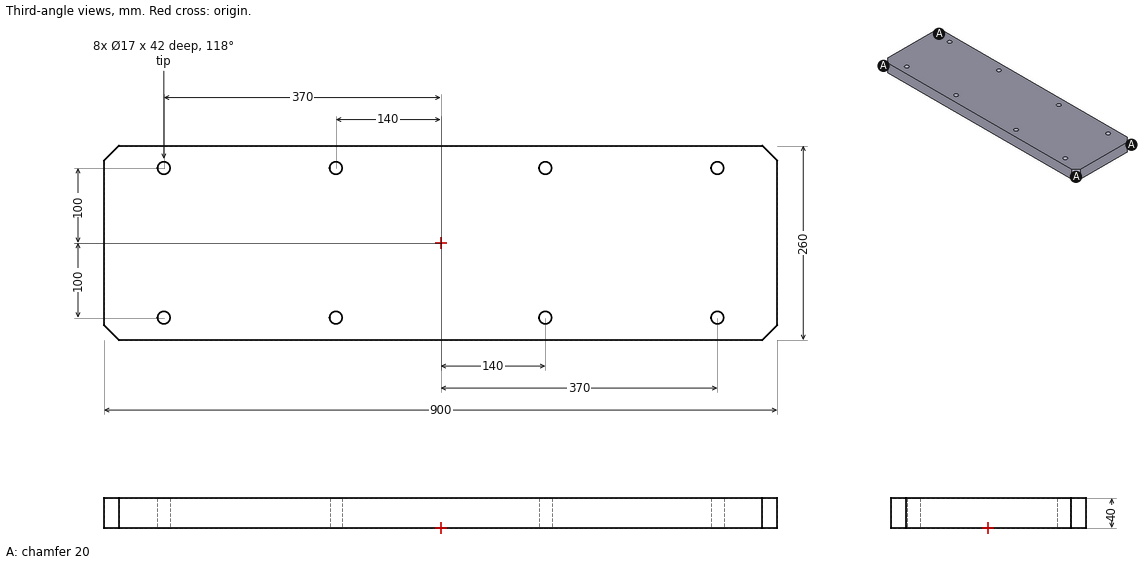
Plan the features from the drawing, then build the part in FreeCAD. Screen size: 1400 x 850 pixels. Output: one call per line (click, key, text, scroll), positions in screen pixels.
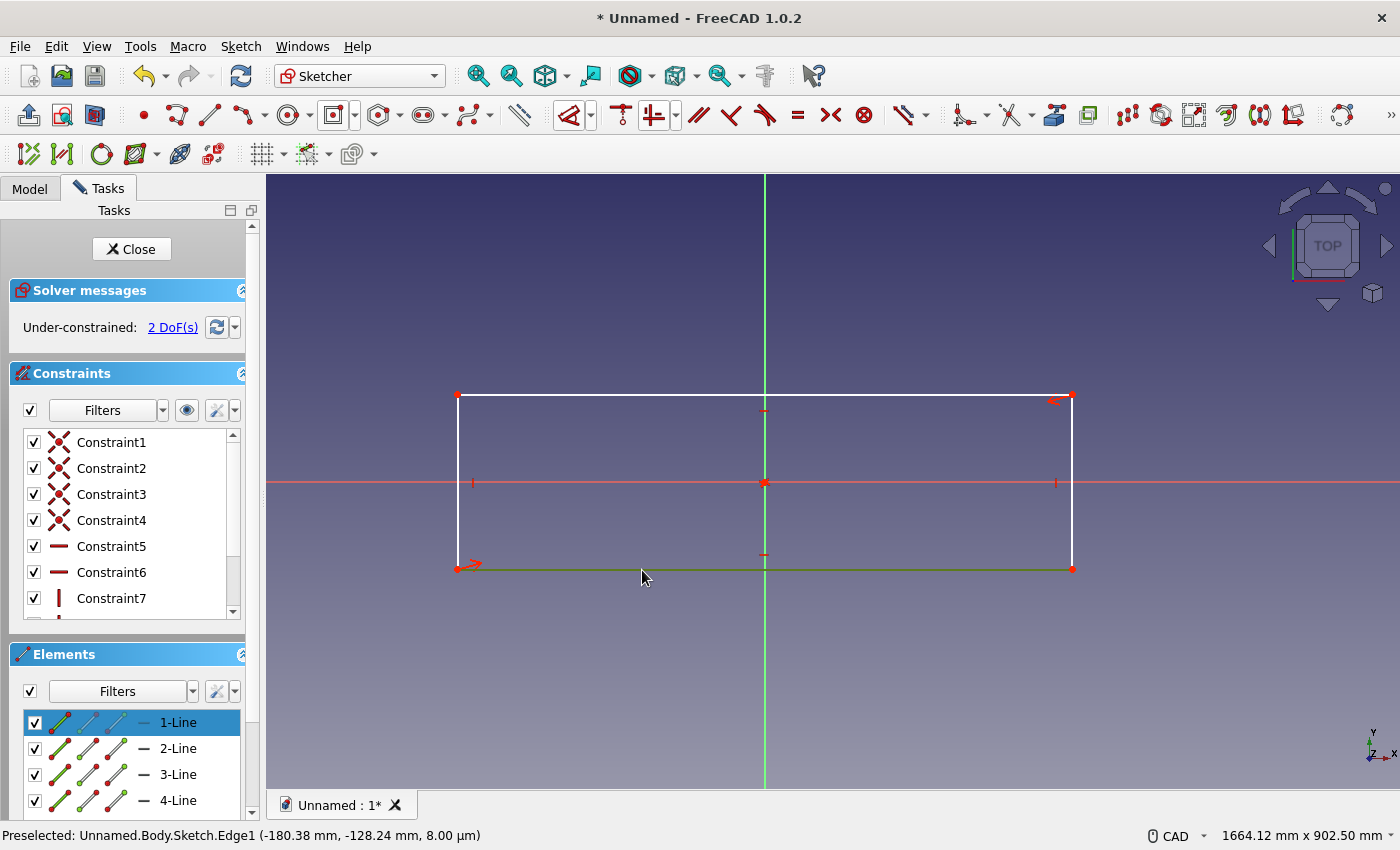
click(590, 116)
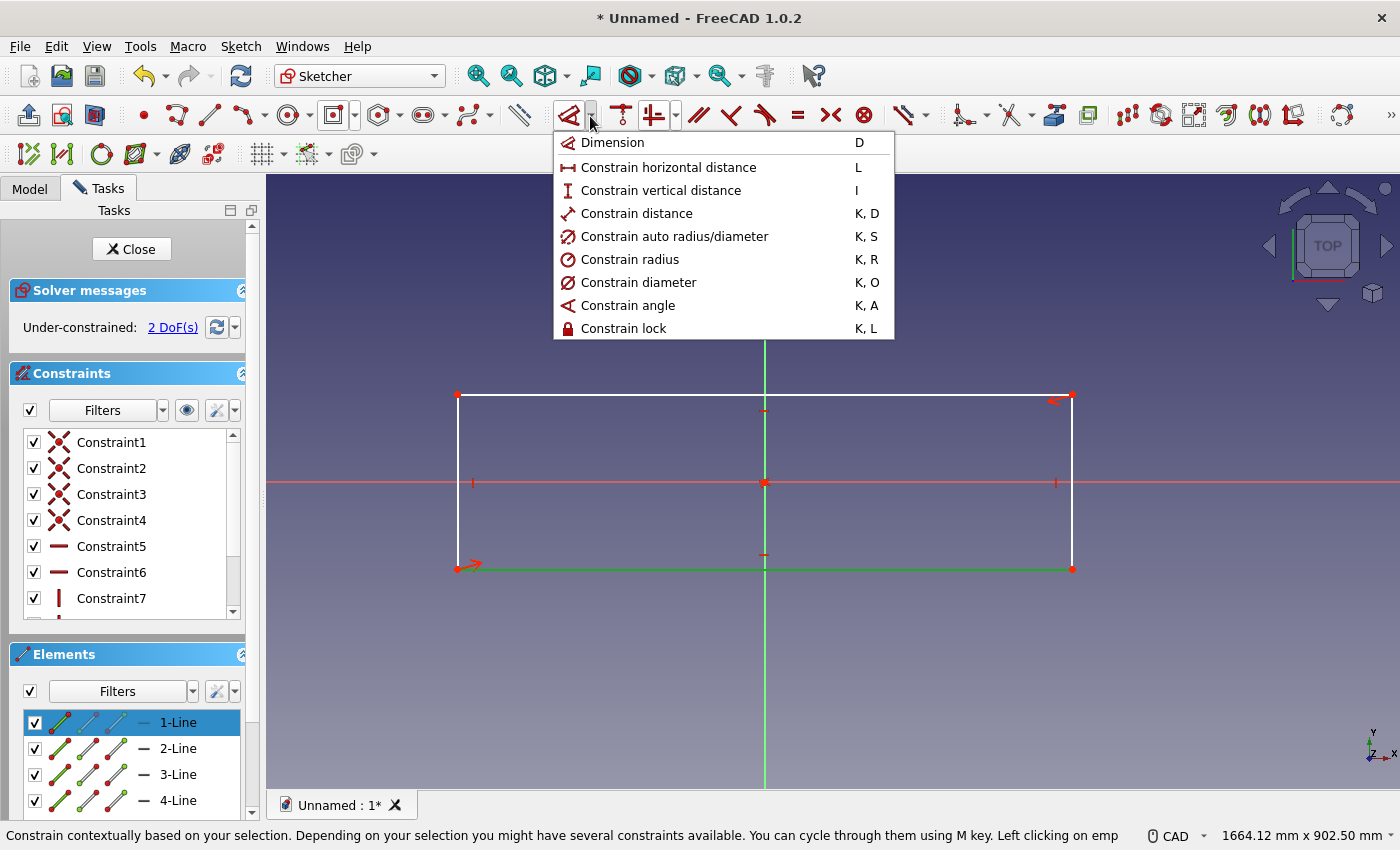
click(724, 168)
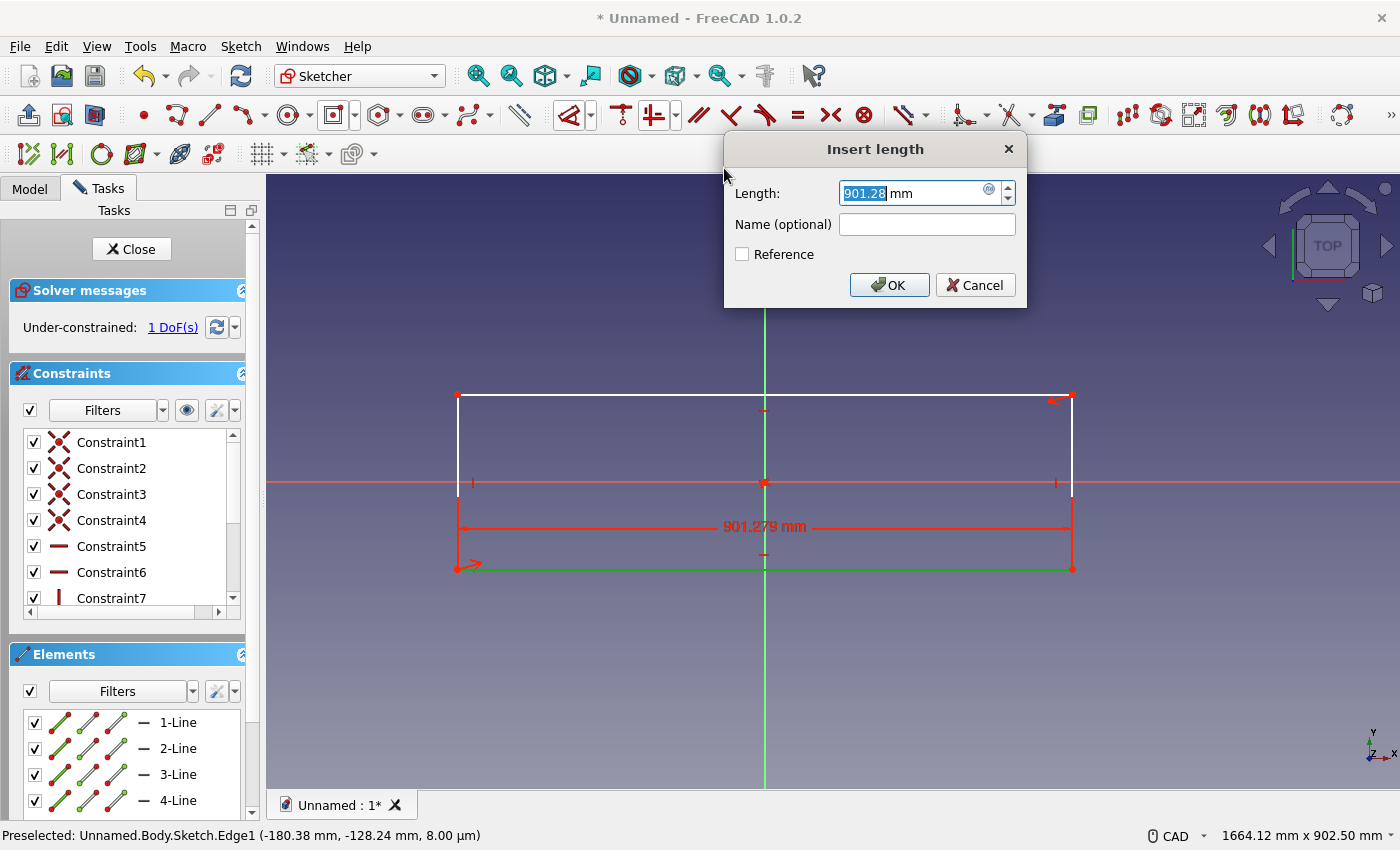
text(900)
key(Return)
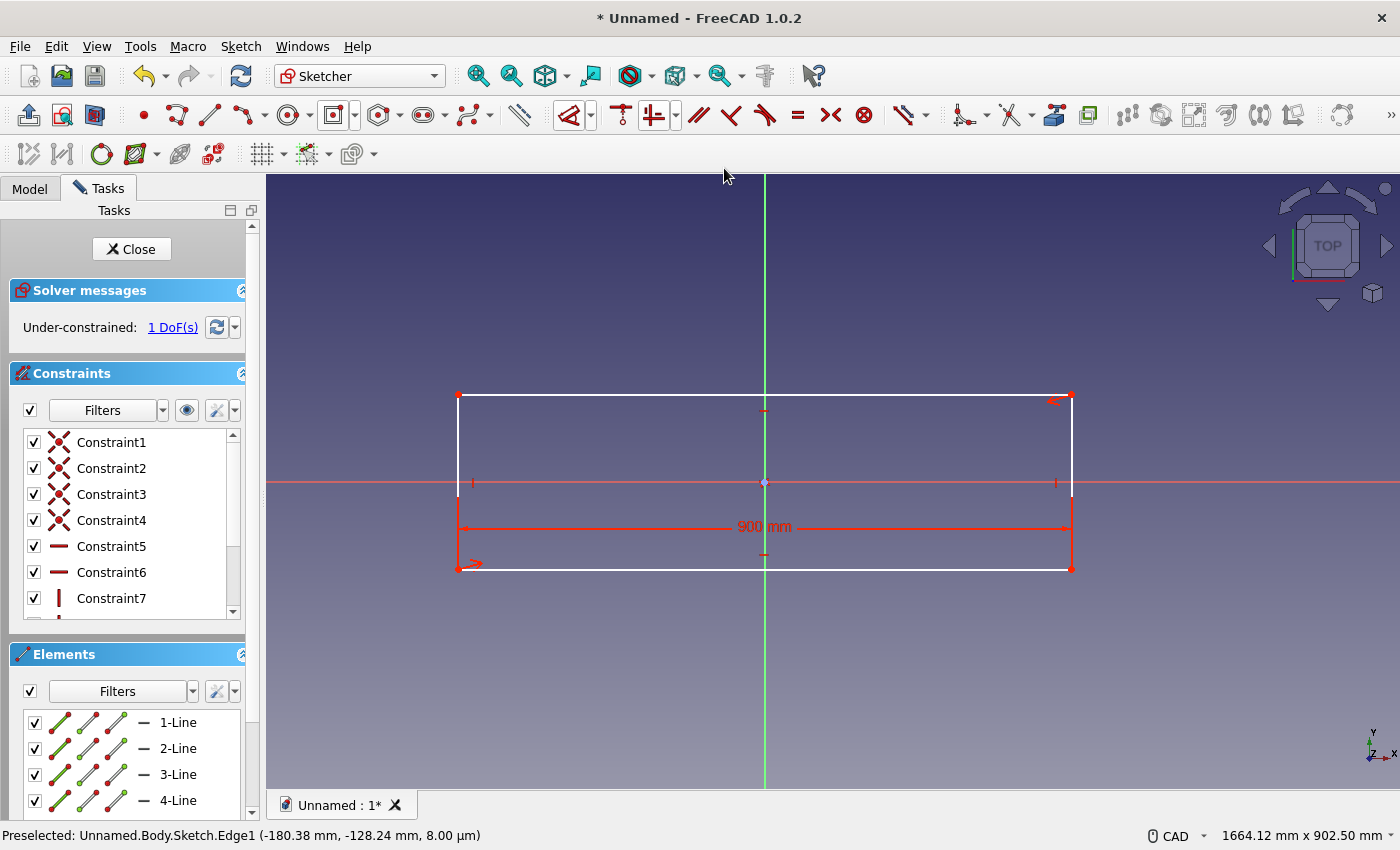
click(1072, 517)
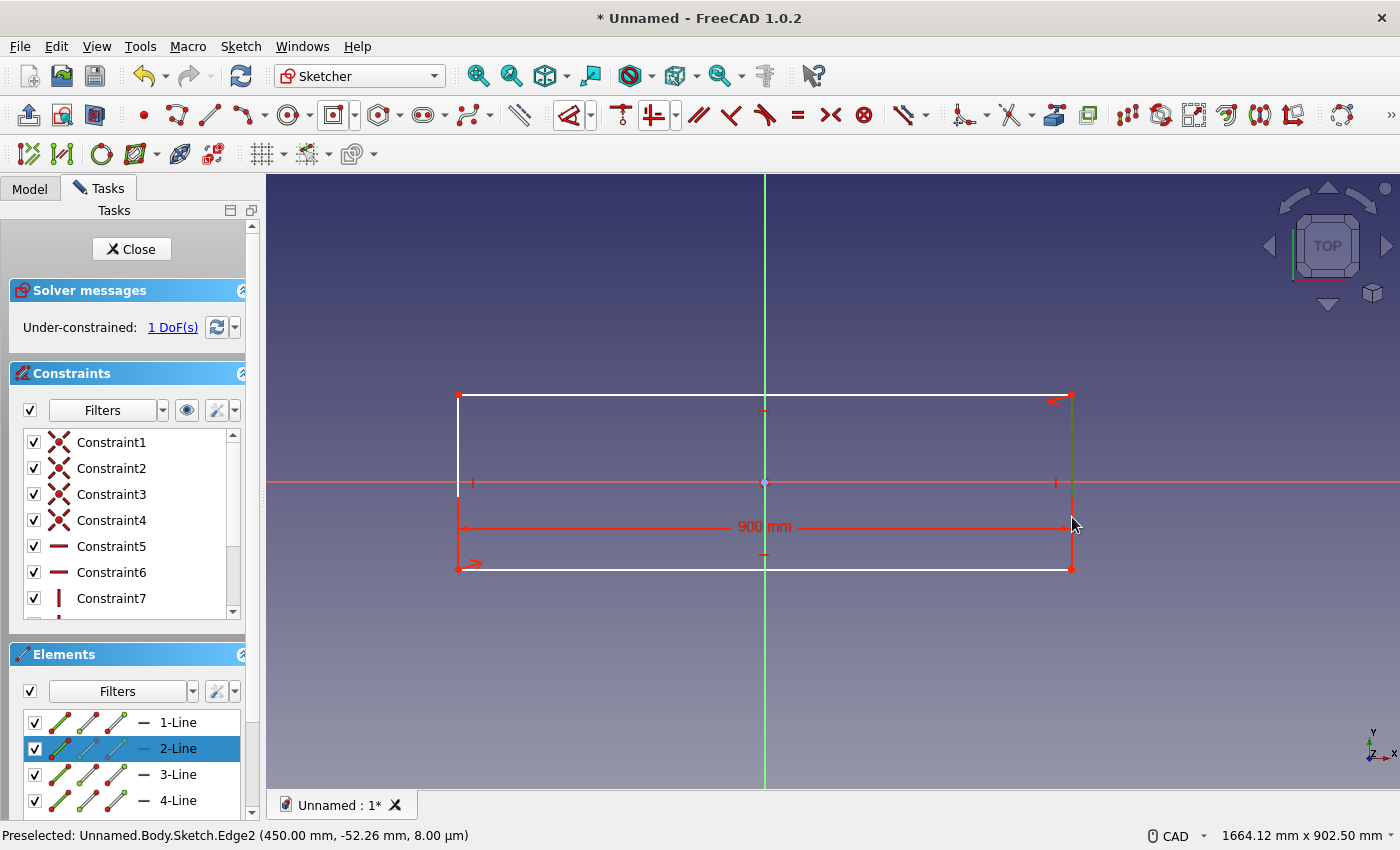
key(i)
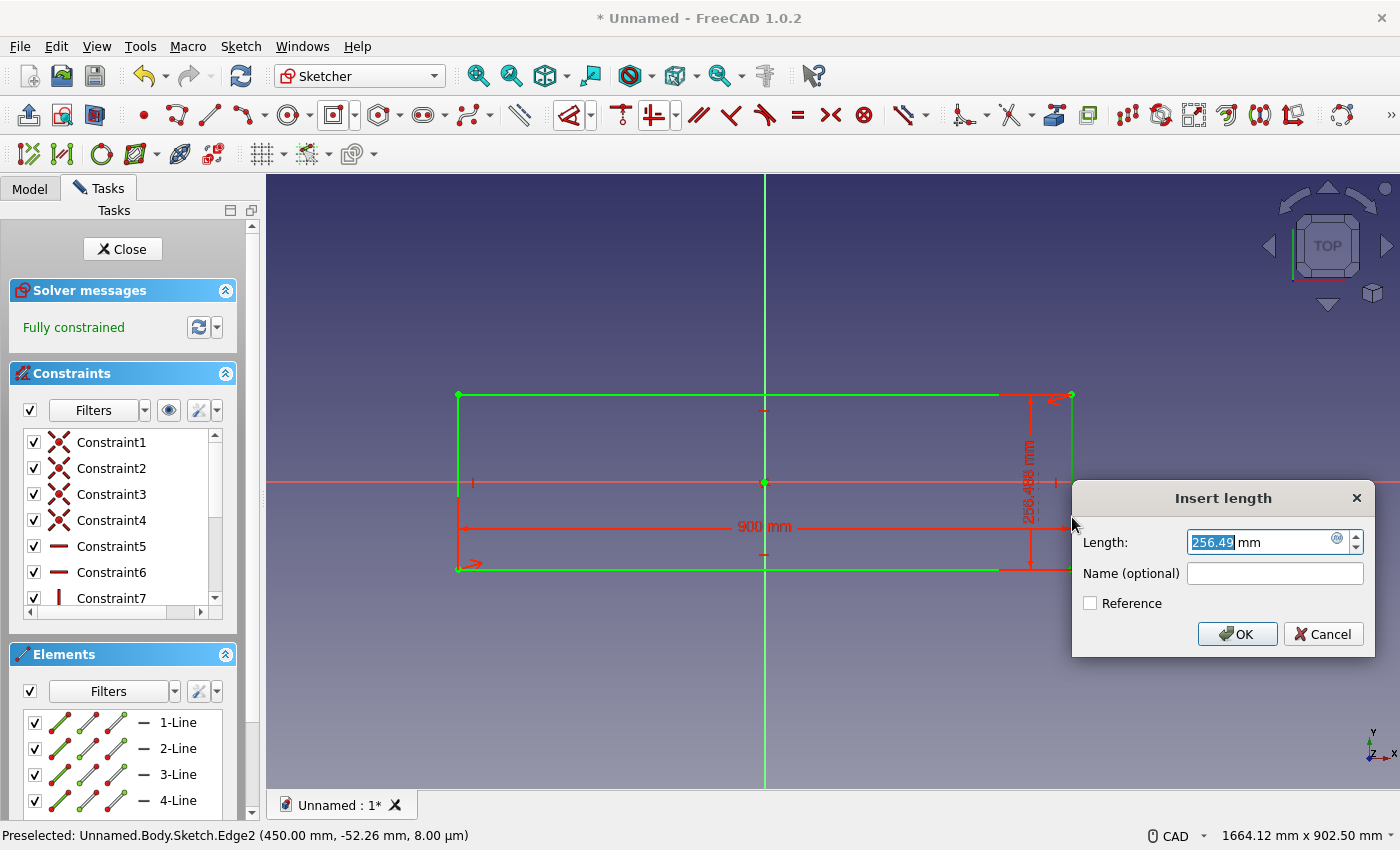
text(260)
key(Return)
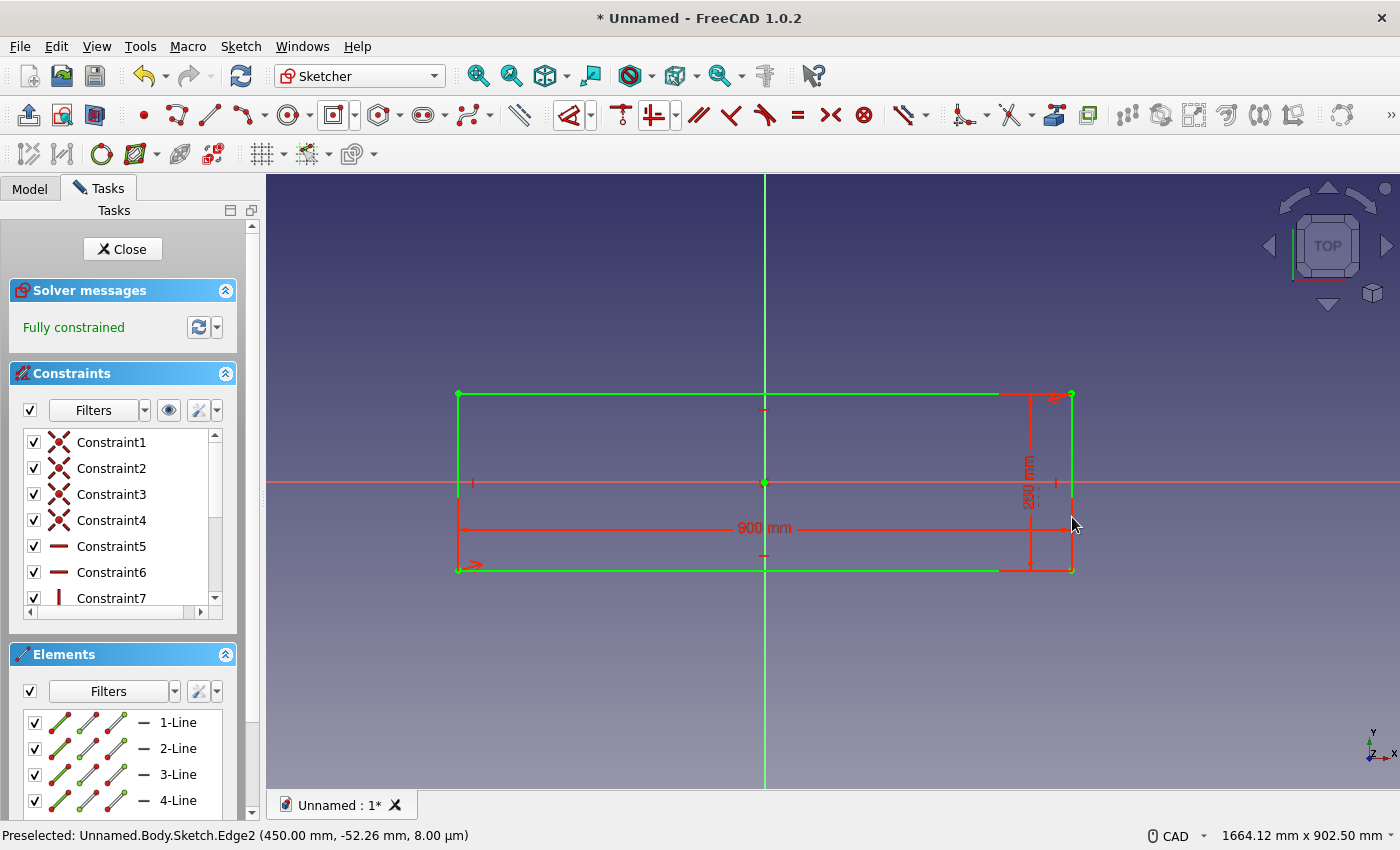
click(123, 249)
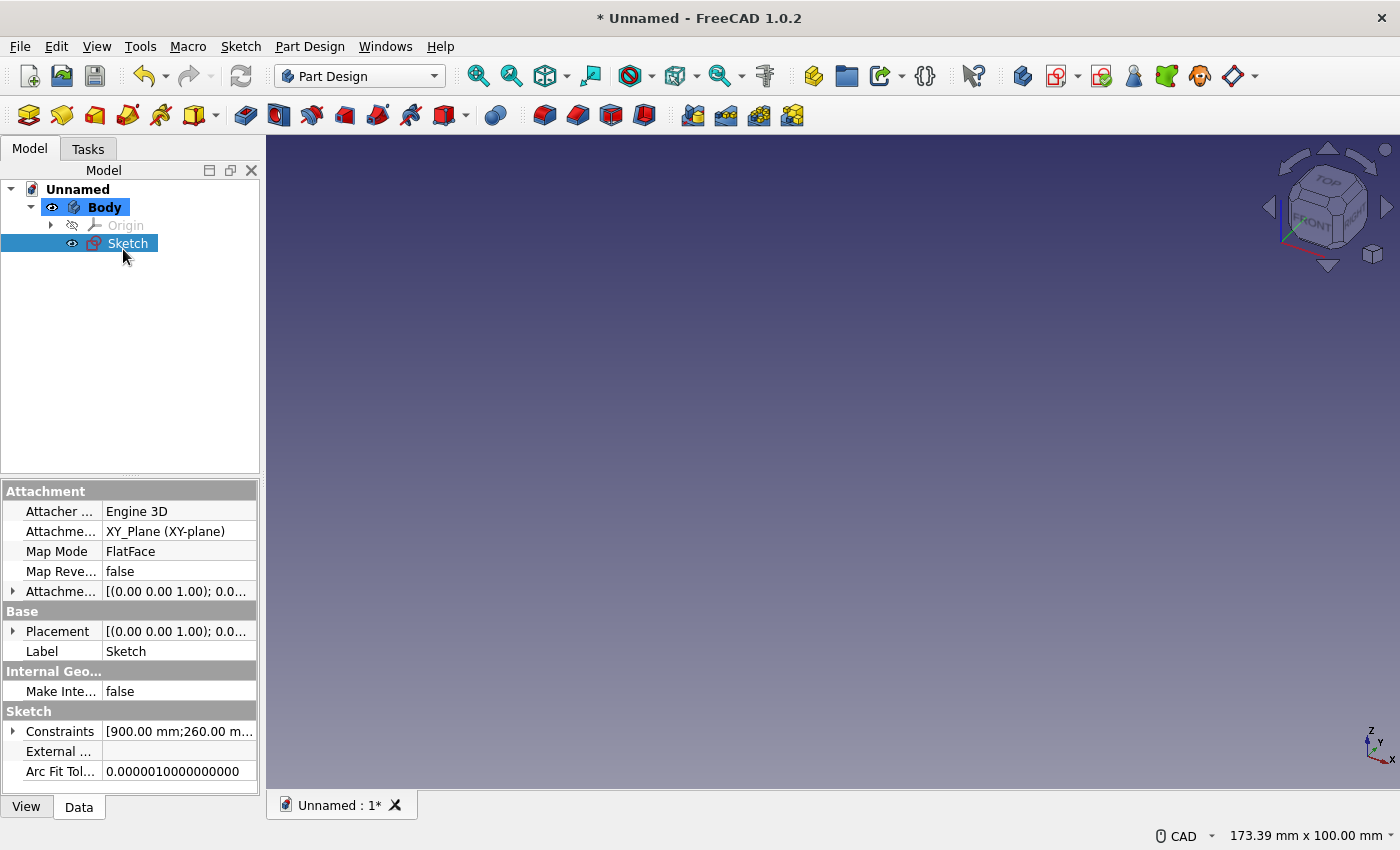
click(29, 116)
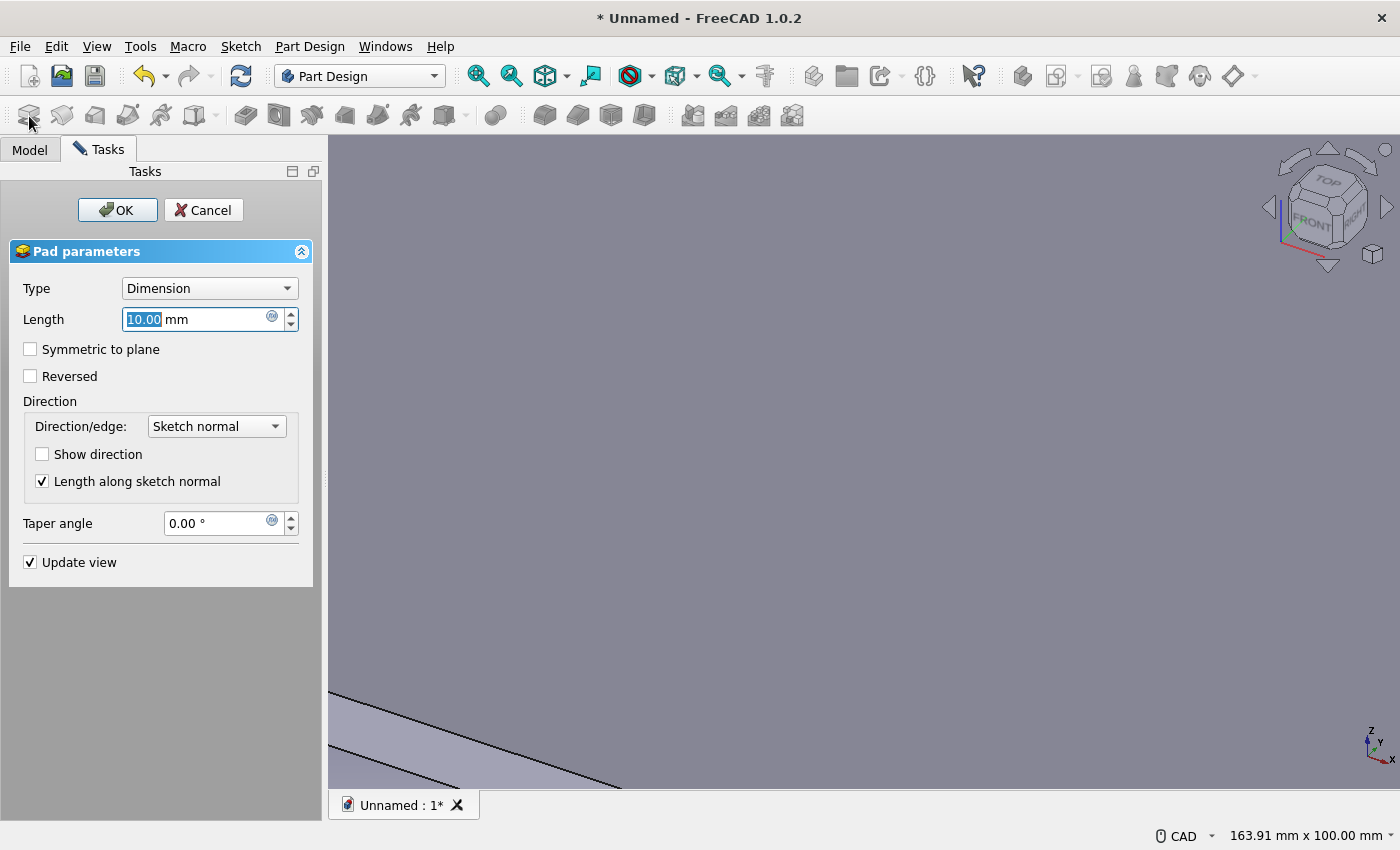
text(40)
key(Tab)